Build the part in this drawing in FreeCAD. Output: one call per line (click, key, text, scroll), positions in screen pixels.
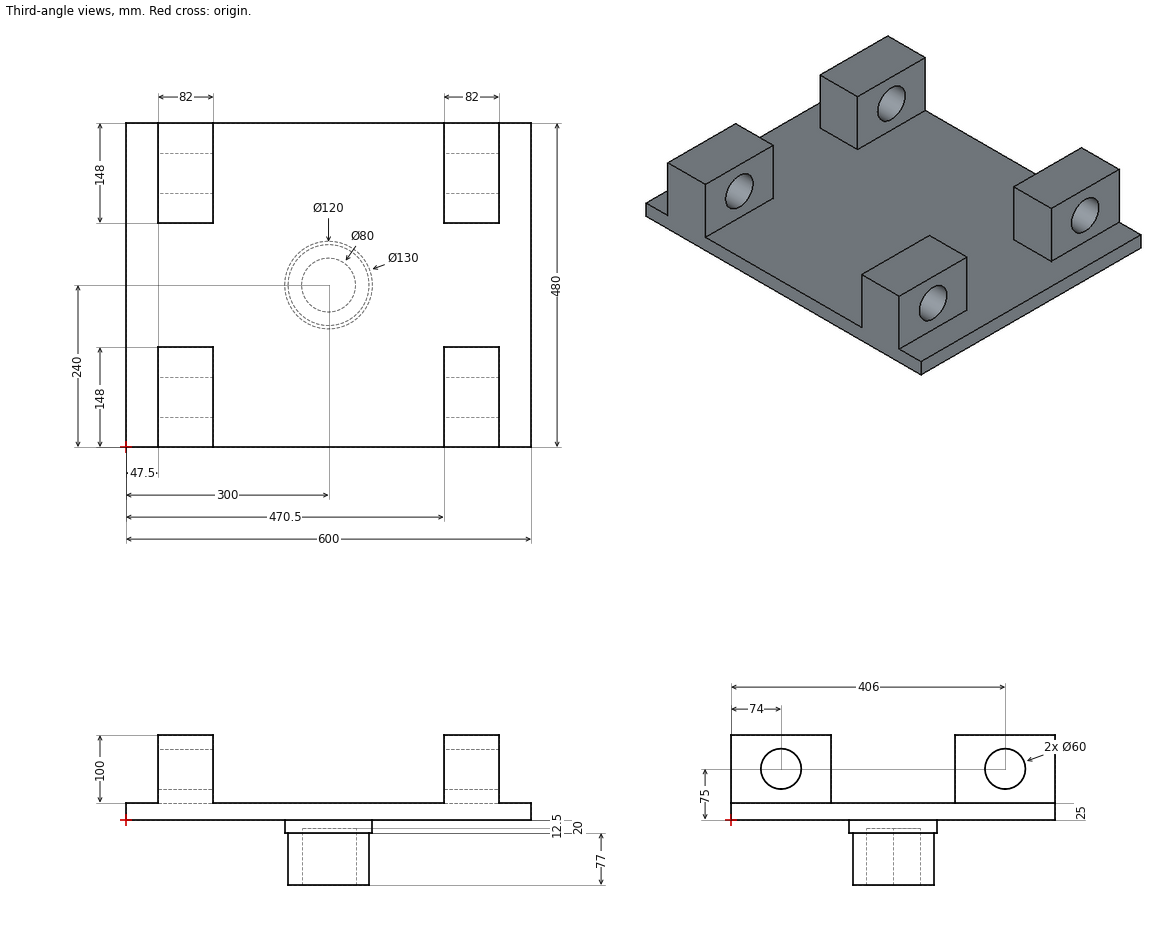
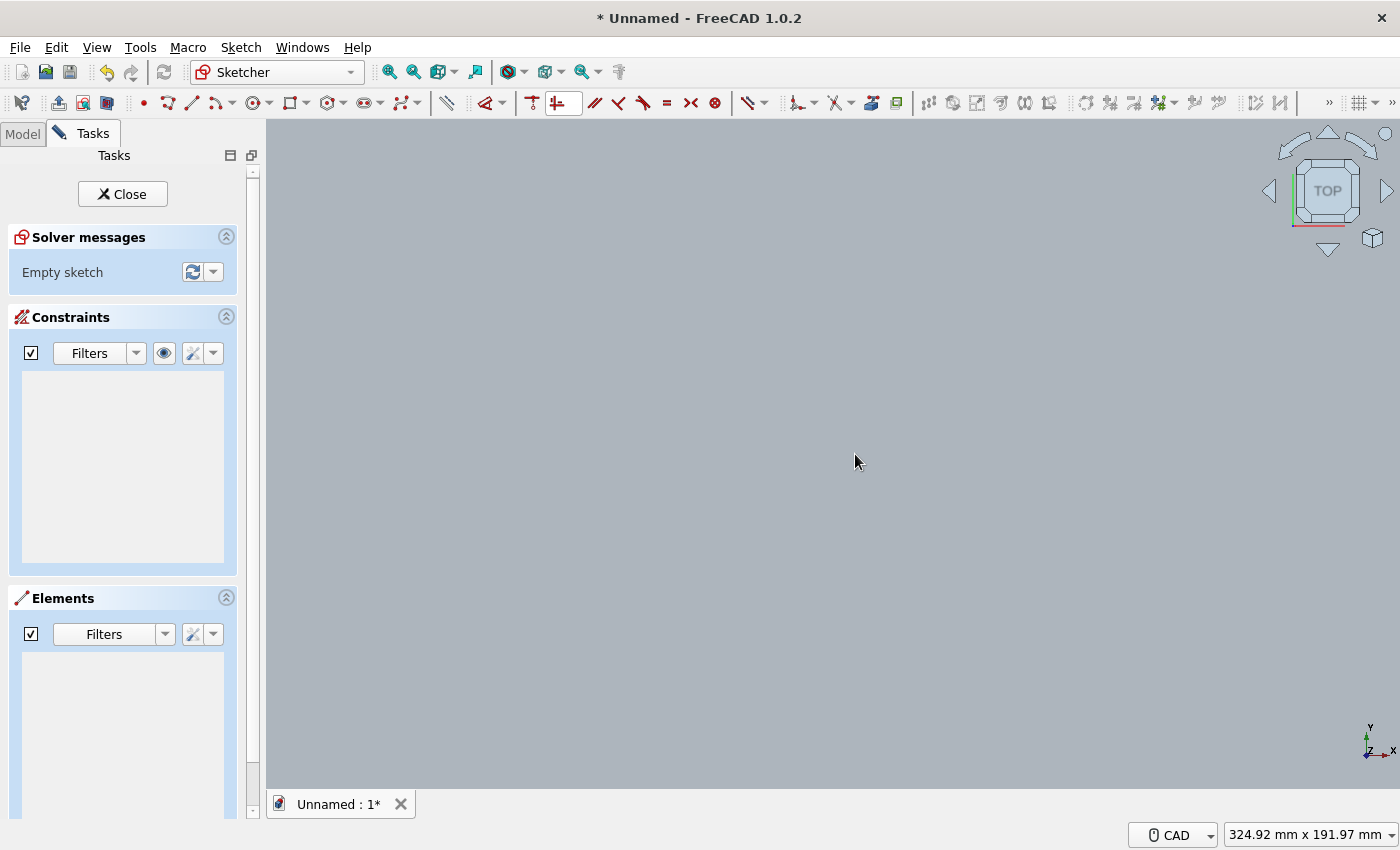
click(254, 104)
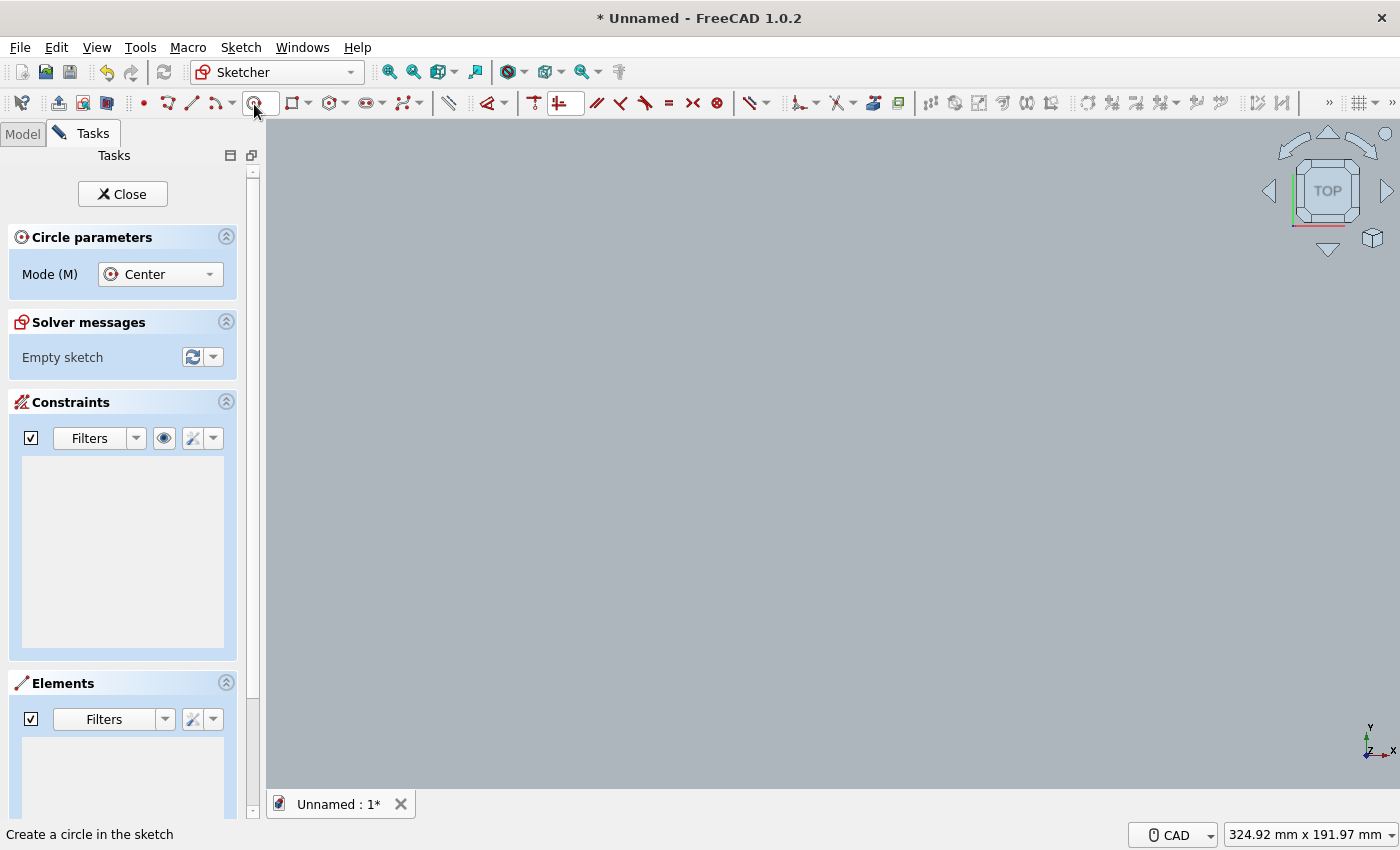
click(764, 452)
move(925, 292)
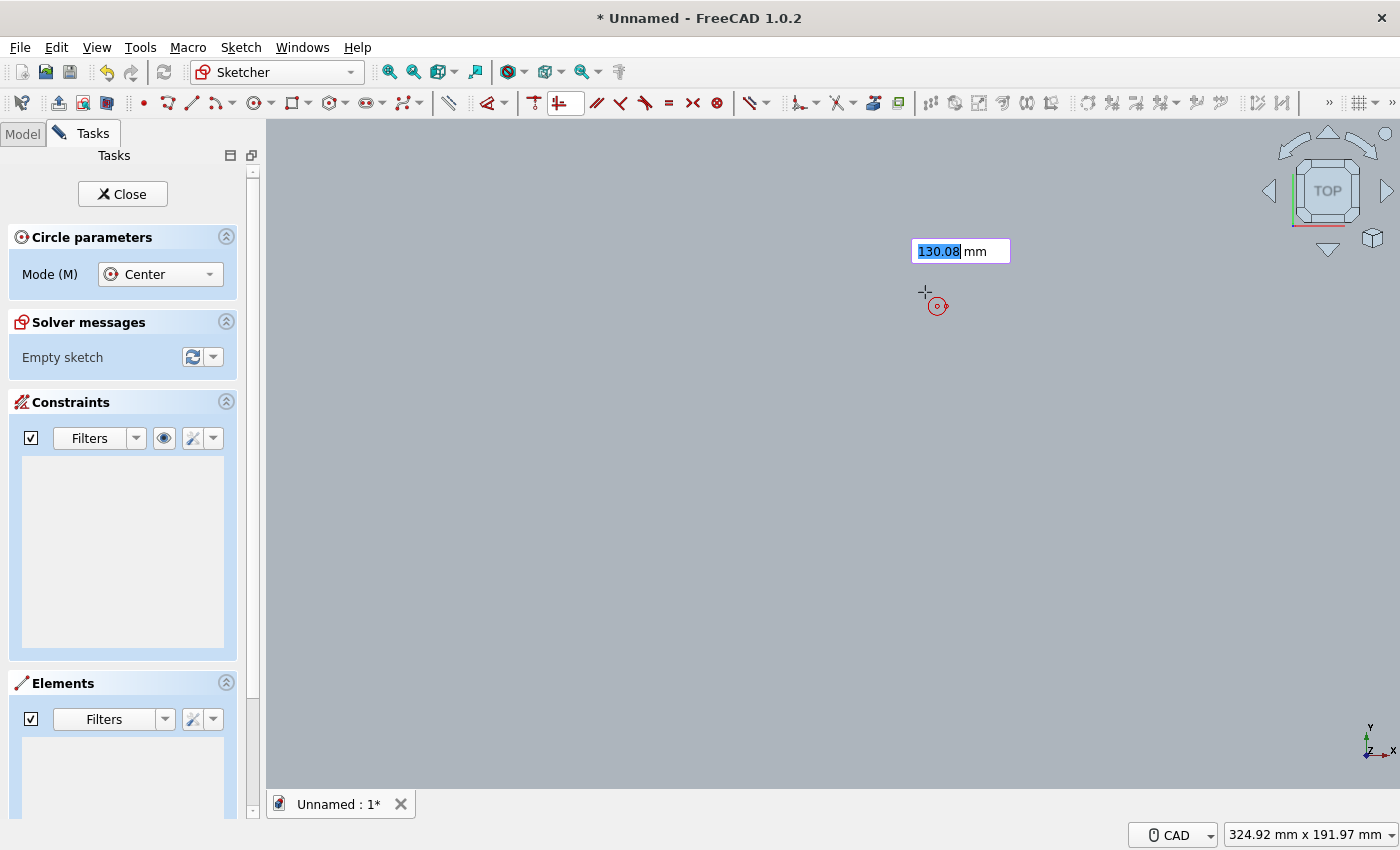
text(130)
key(Return)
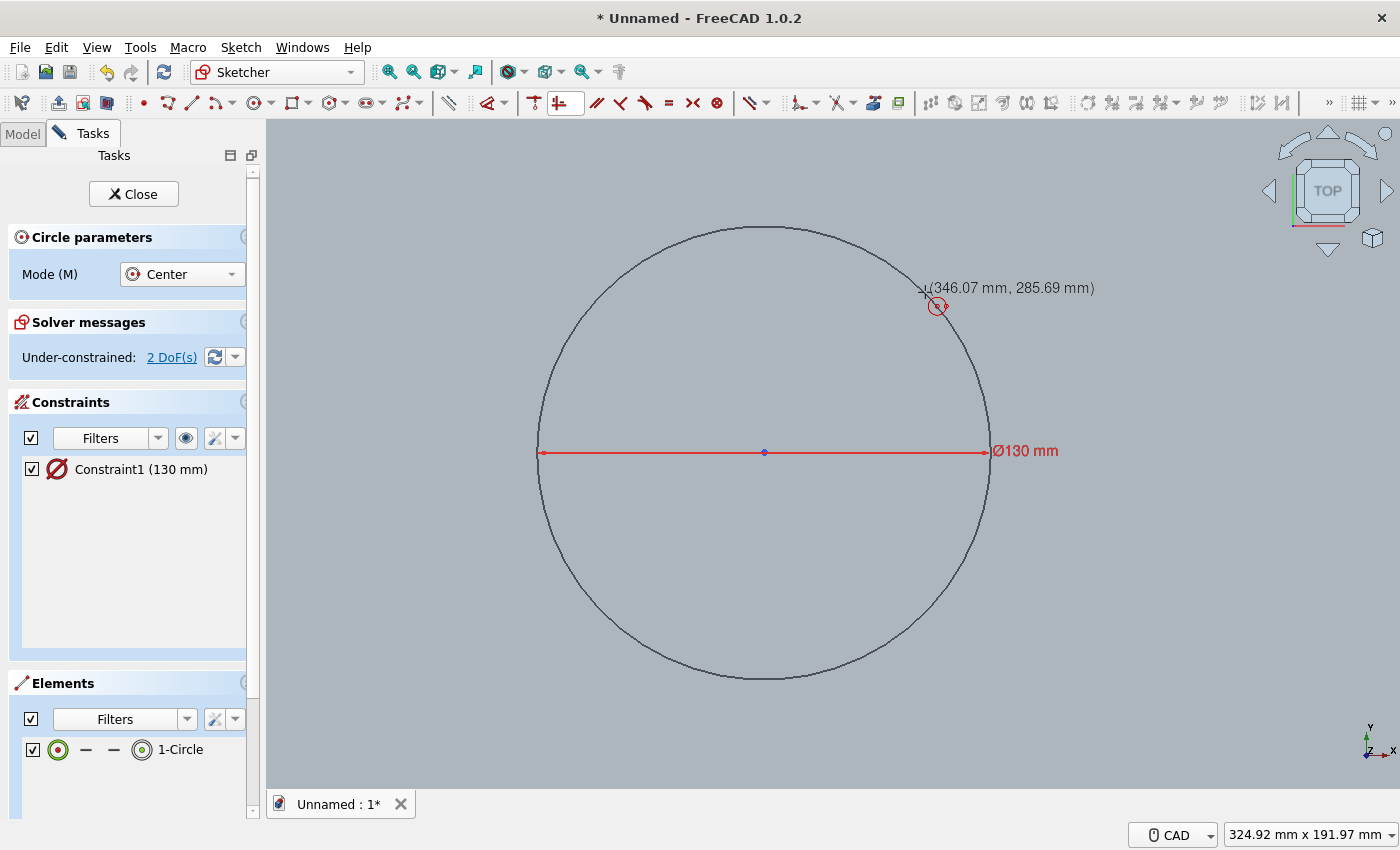
click(764, 453)
move(863, 354)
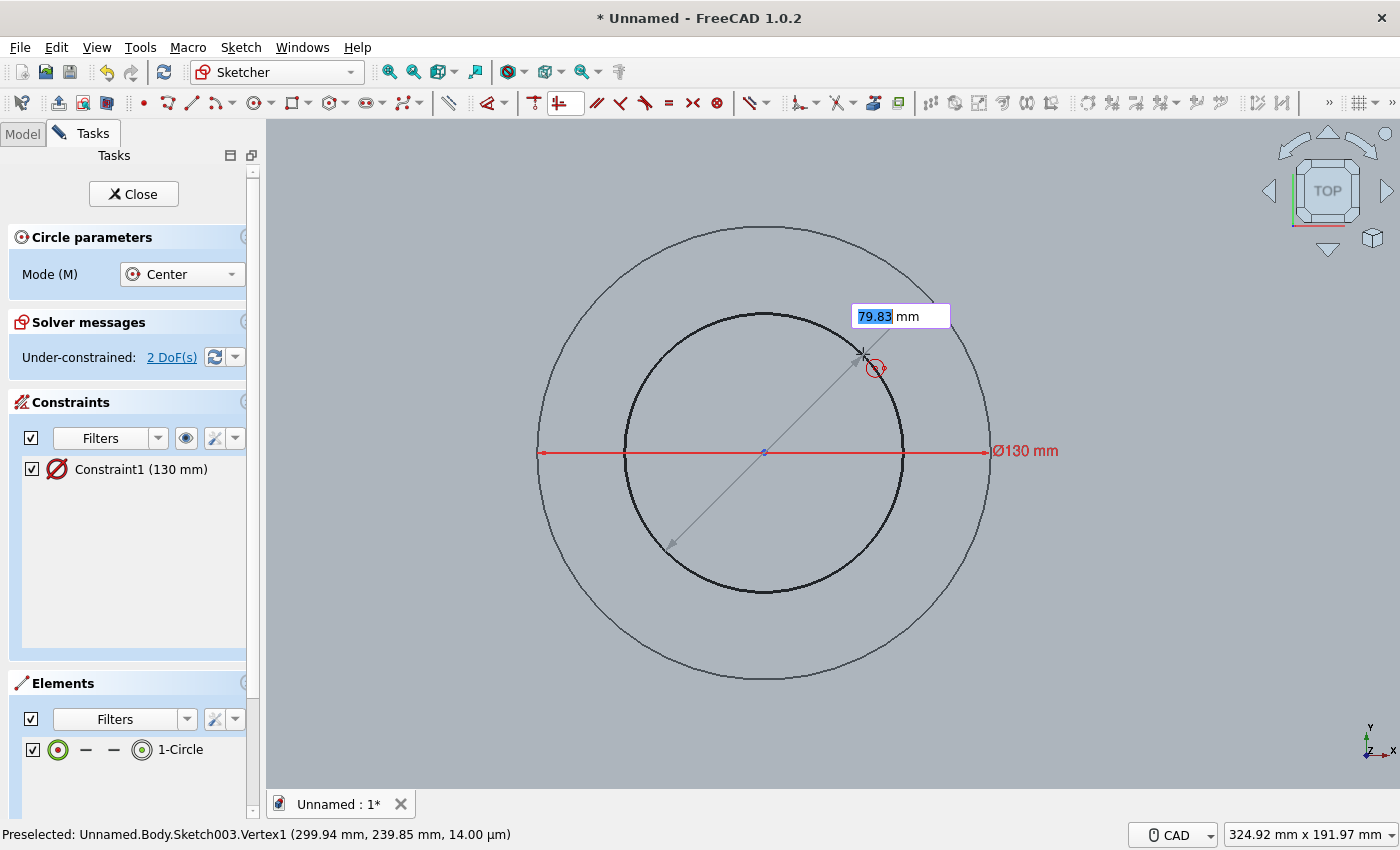
text(80)
key(Return)
key(Escape)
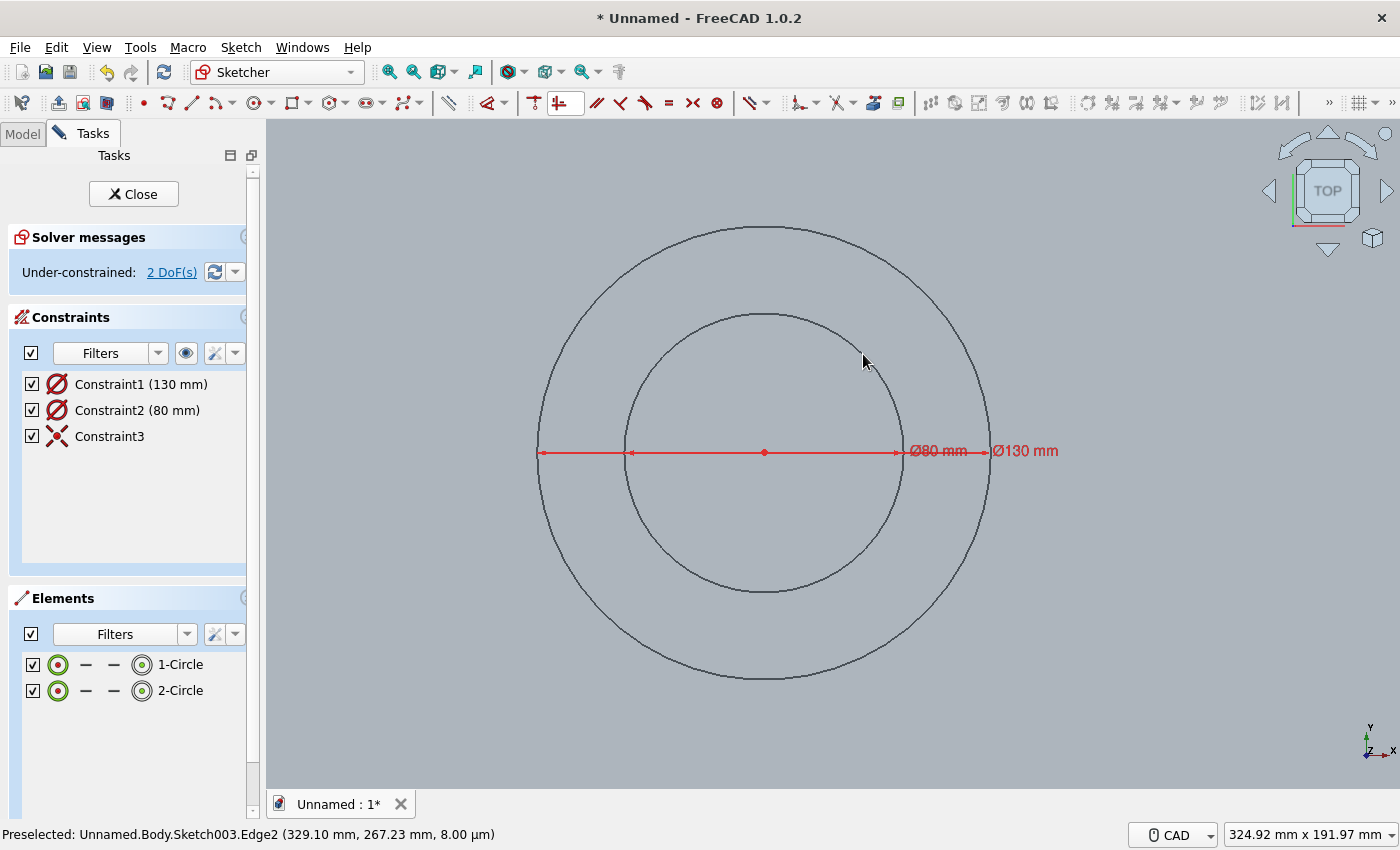
click(488, 104)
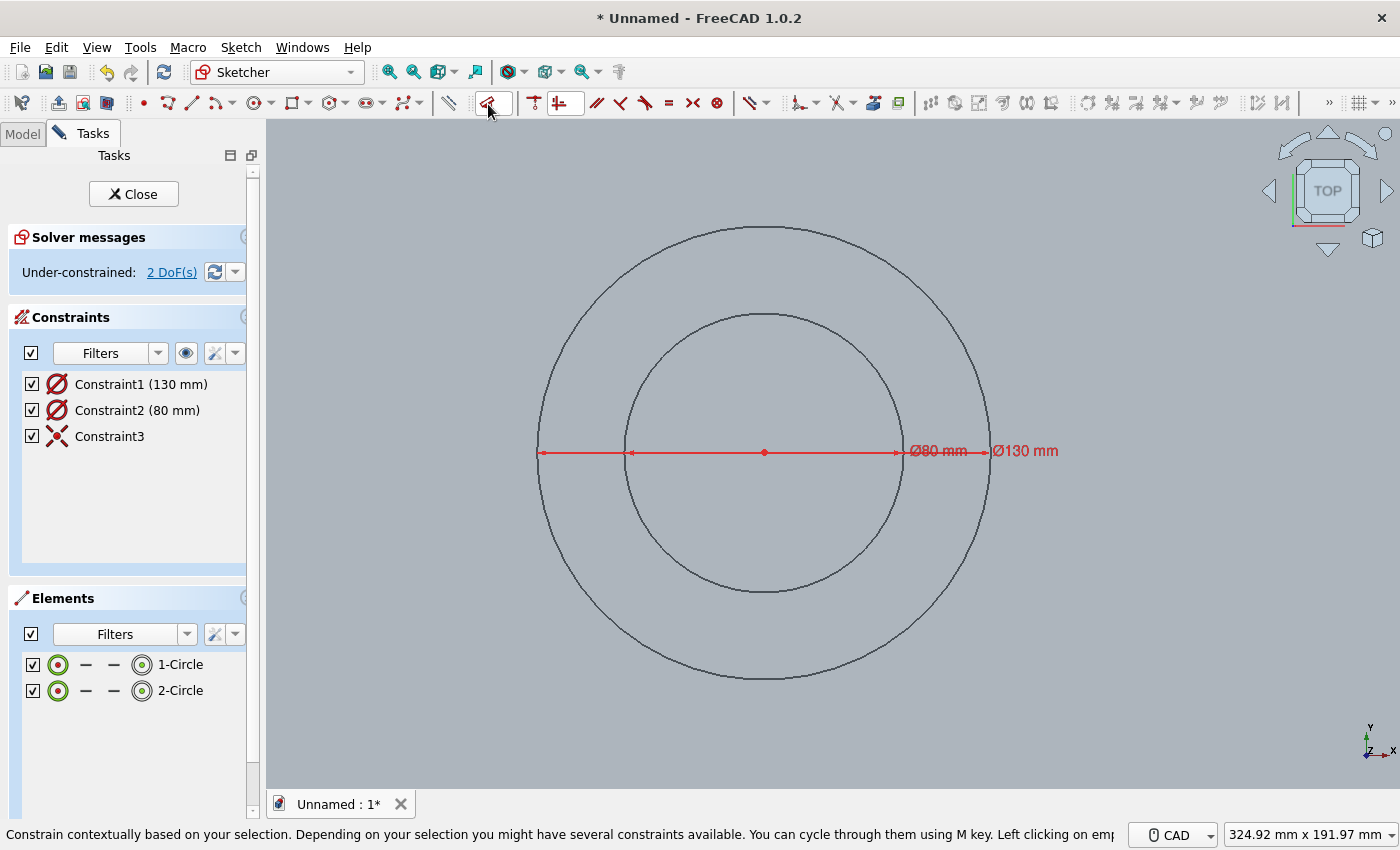
click(764, 453)
click(421, 419)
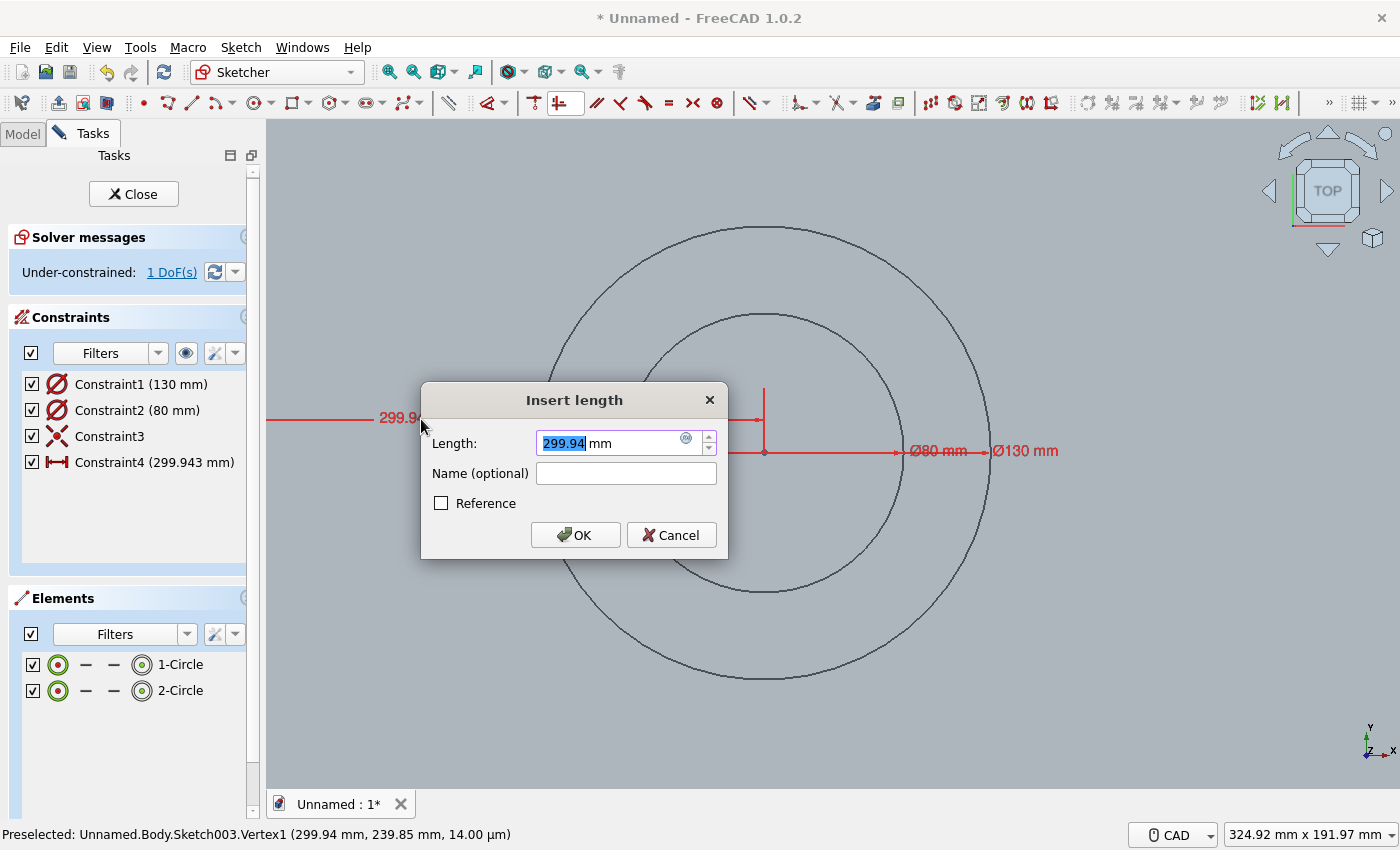
text(300)
key(Return)